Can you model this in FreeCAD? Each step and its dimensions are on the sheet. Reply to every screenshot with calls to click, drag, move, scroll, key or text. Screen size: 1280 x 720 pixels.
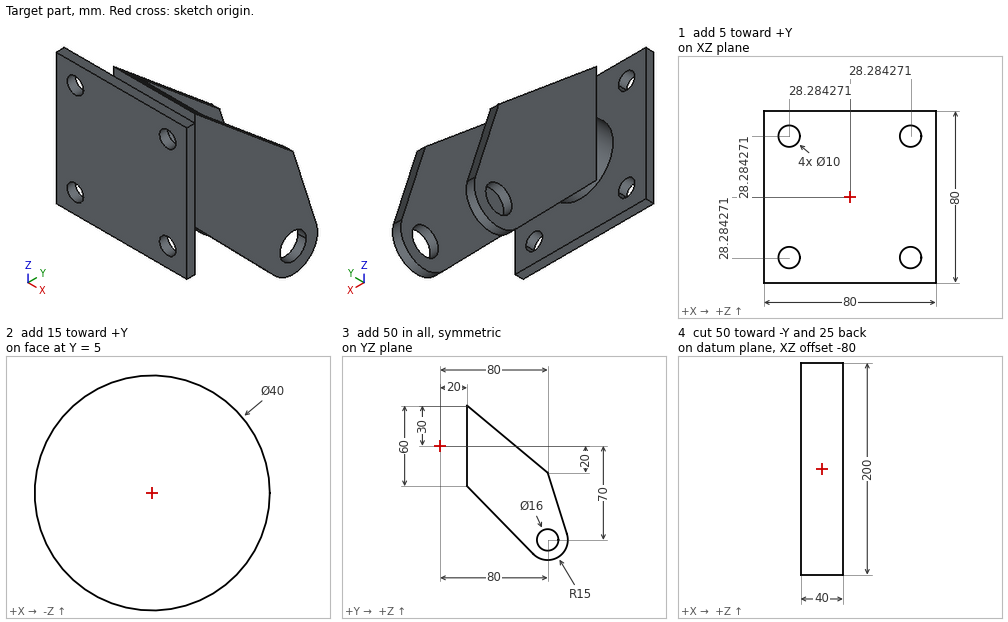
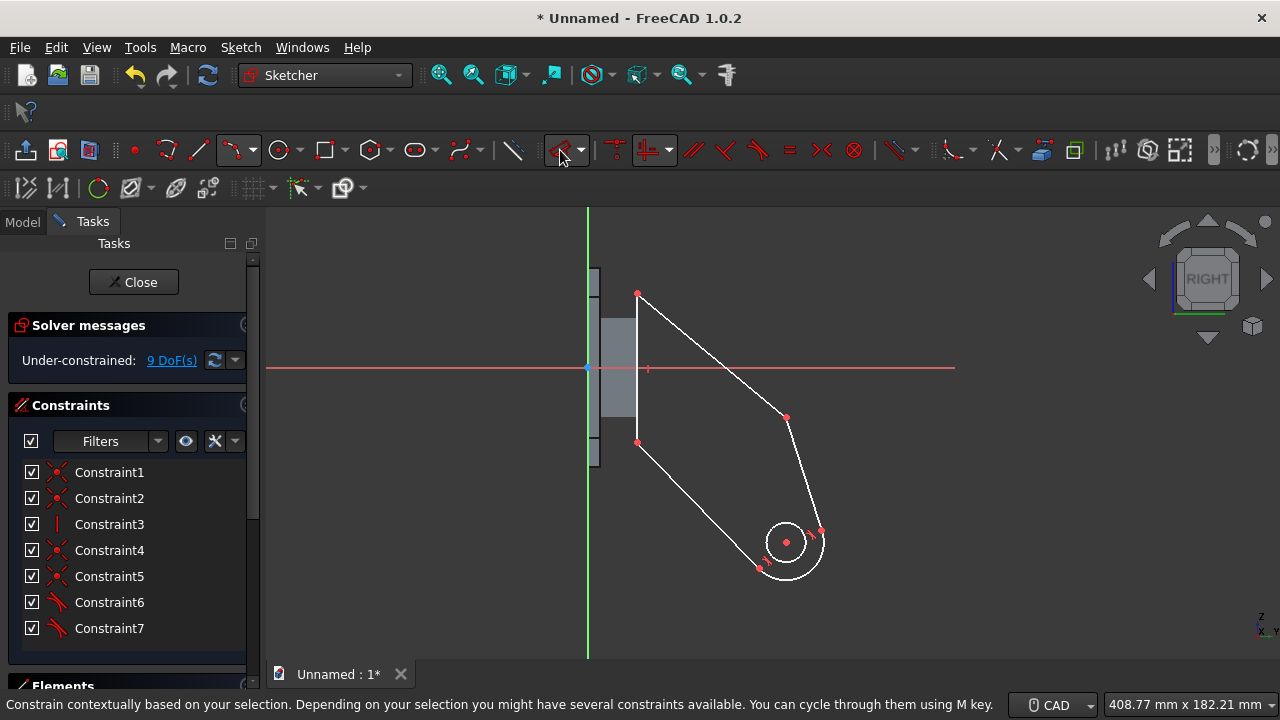
click(786, 580)
click(786, 612)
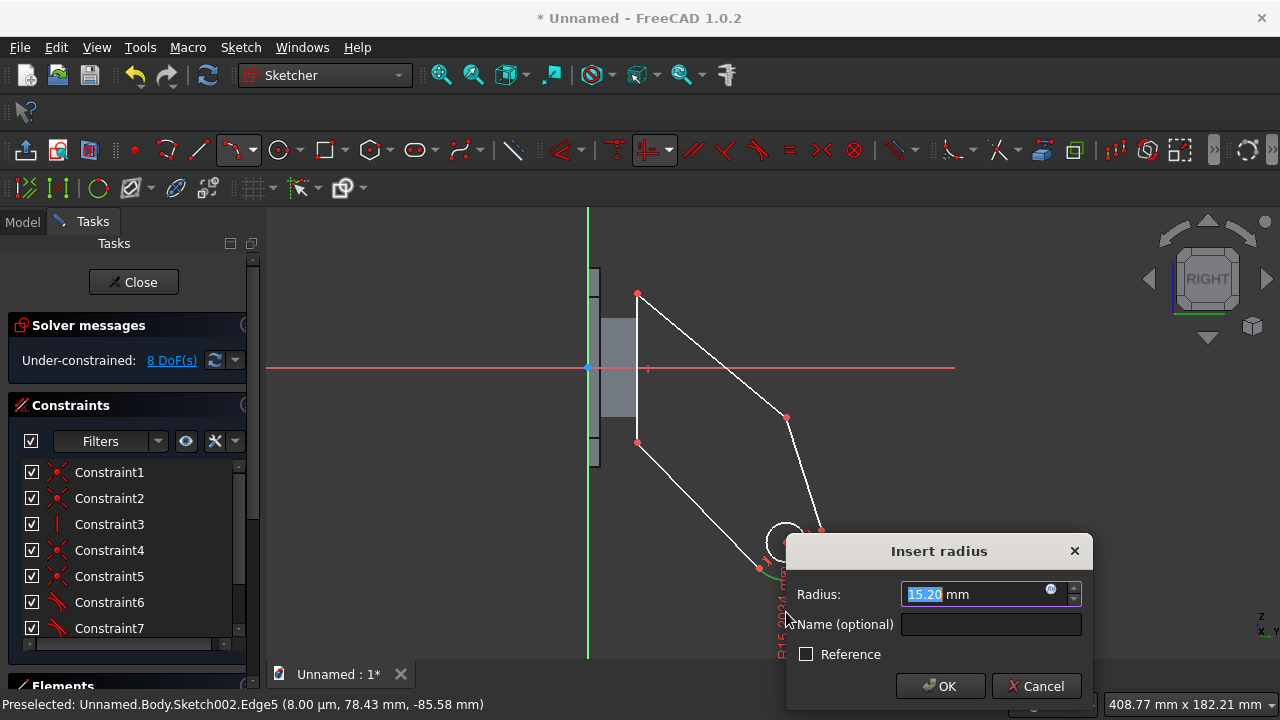
text(15)
key(Return)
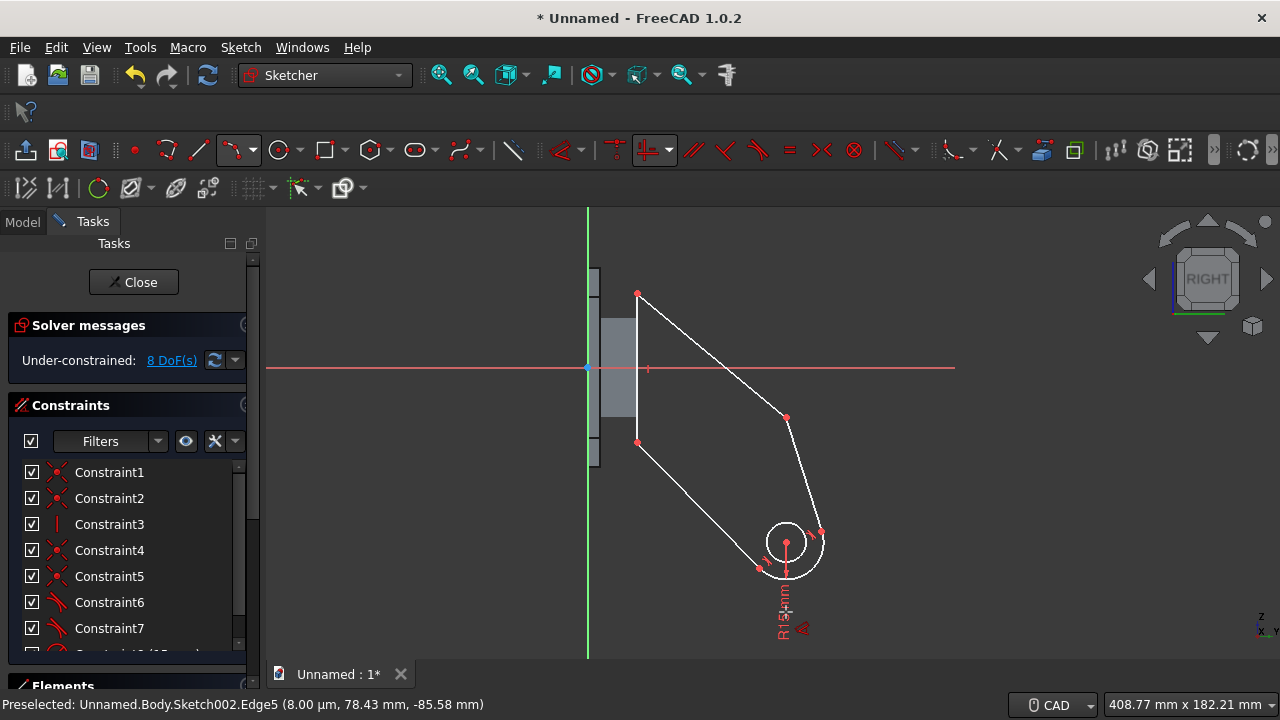
click(800, 528)
click(836, 527)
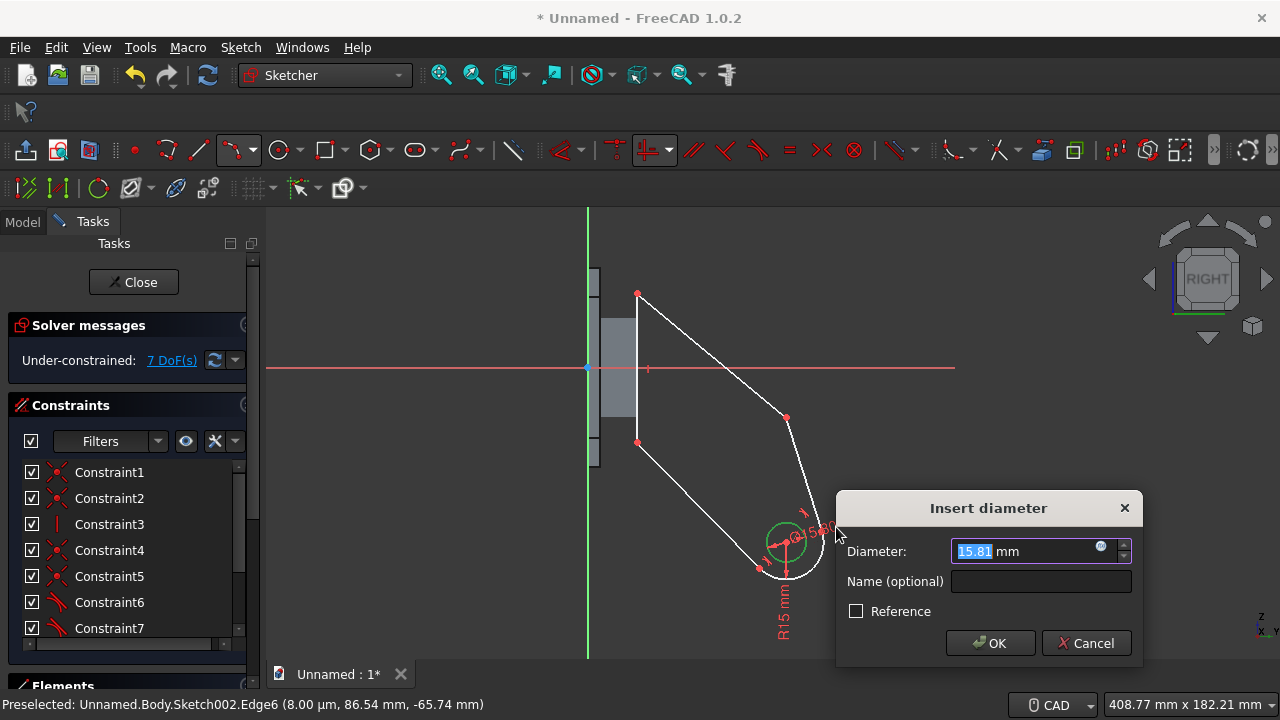
text(16)
key(Return)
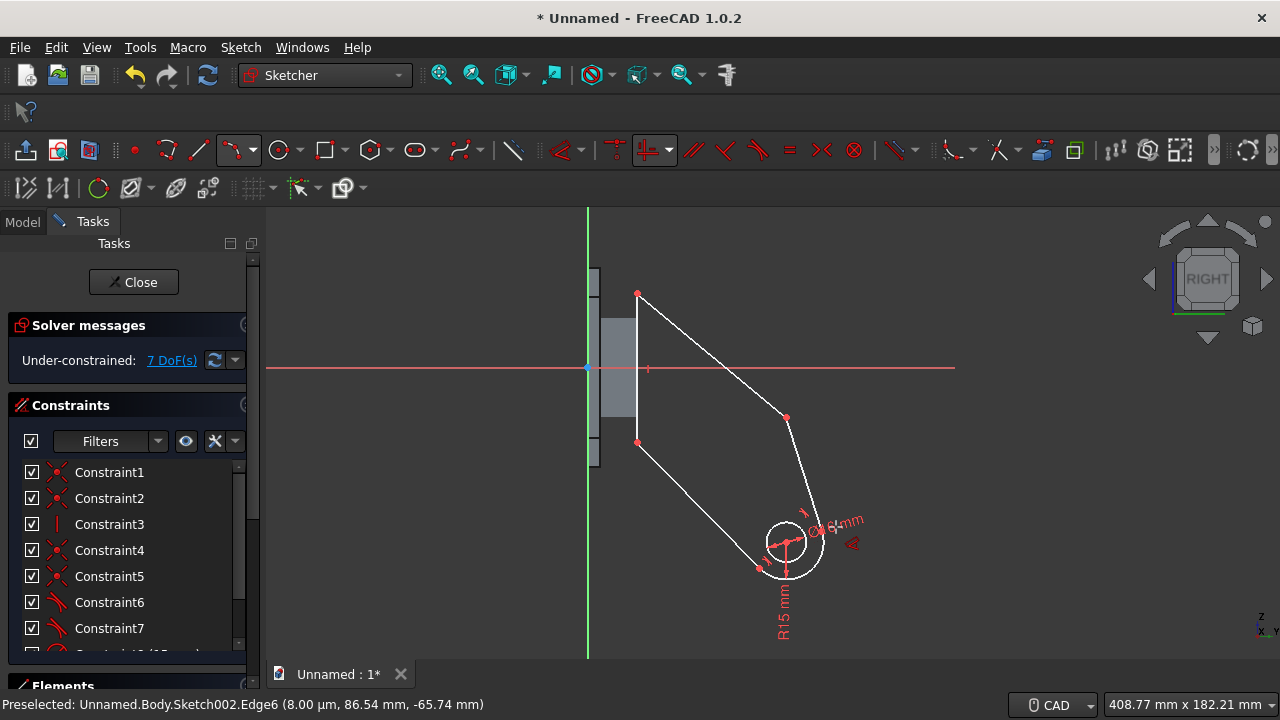
click(637, 339)
click(603, 334)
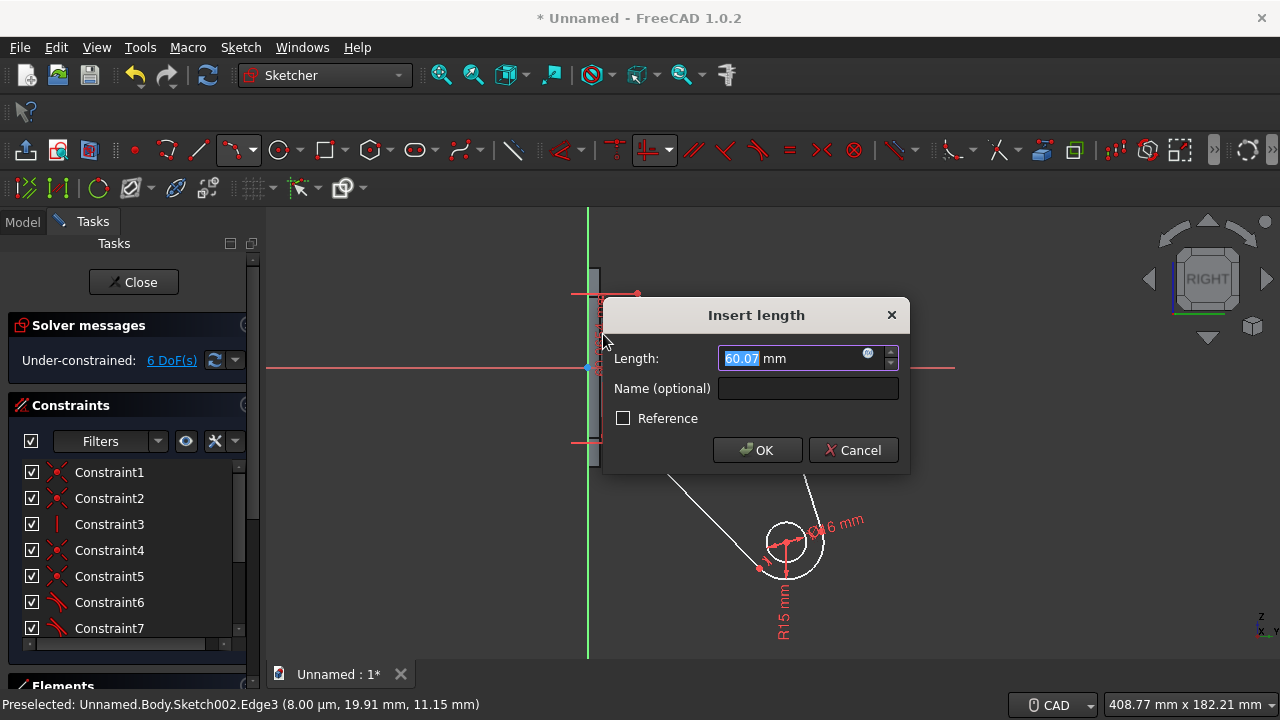
text(60)
key(Return)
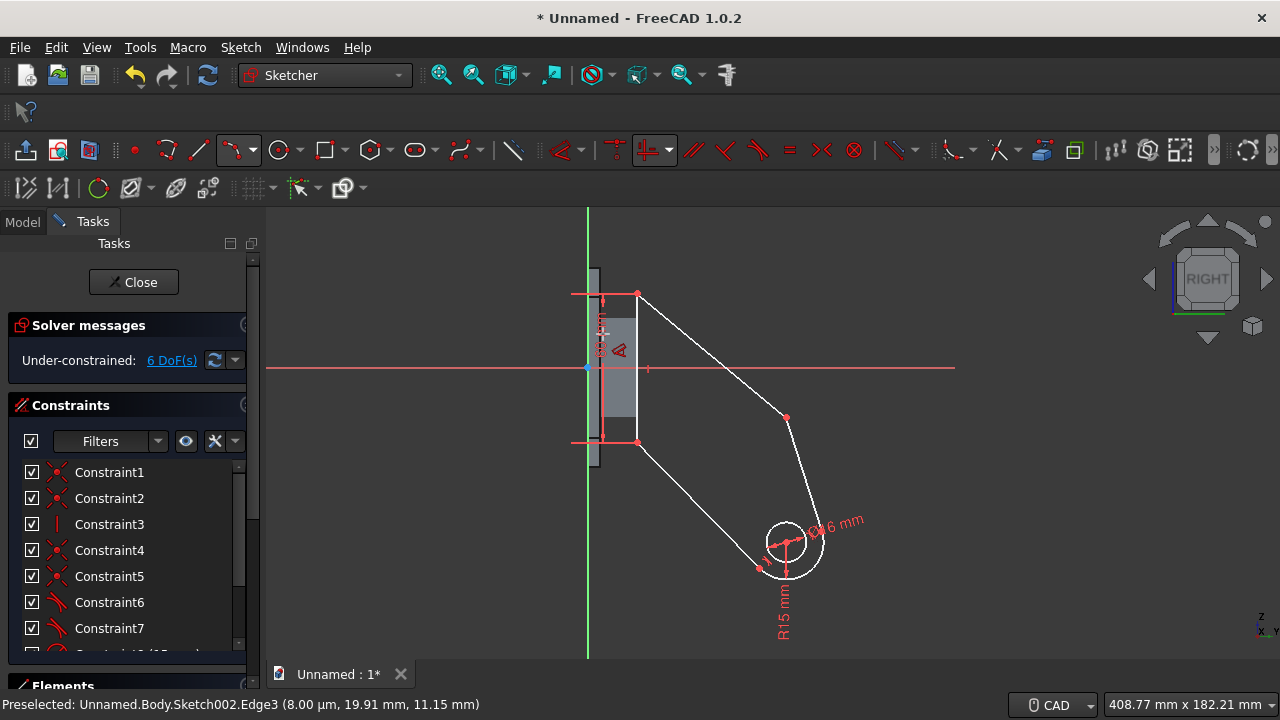
click(786, 542)
click(687, 576)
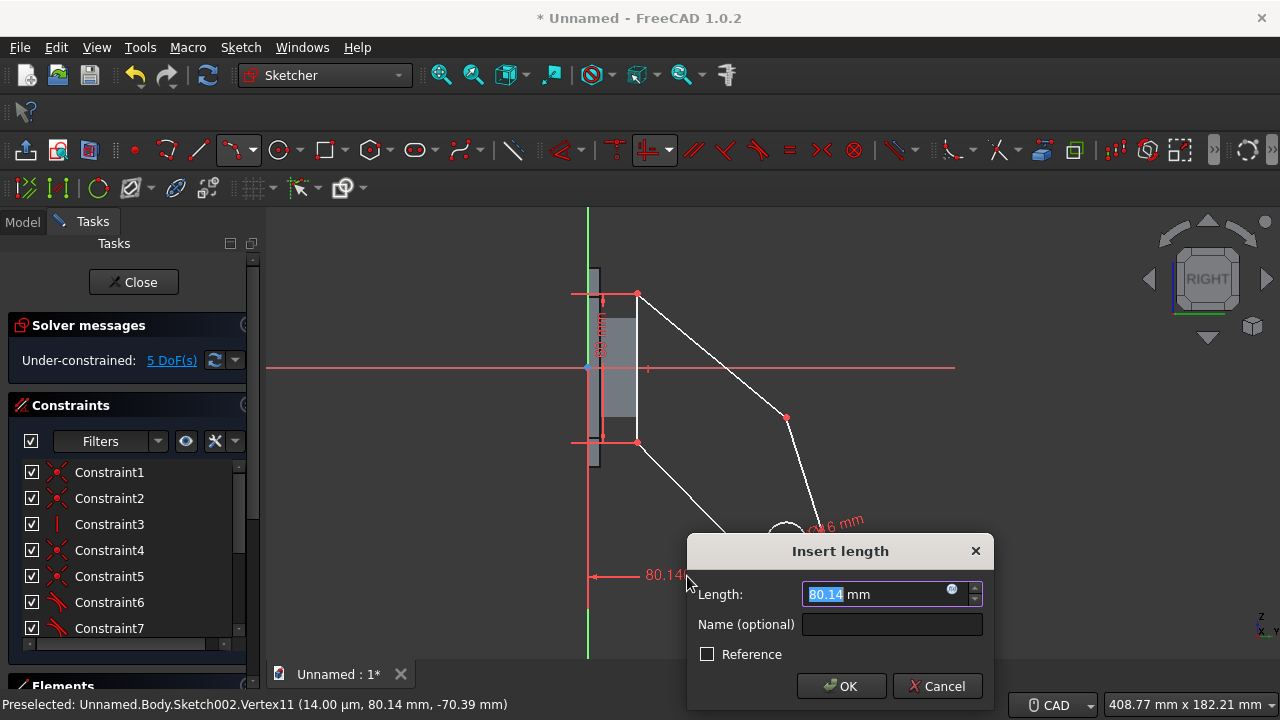
text(80)
key(Return)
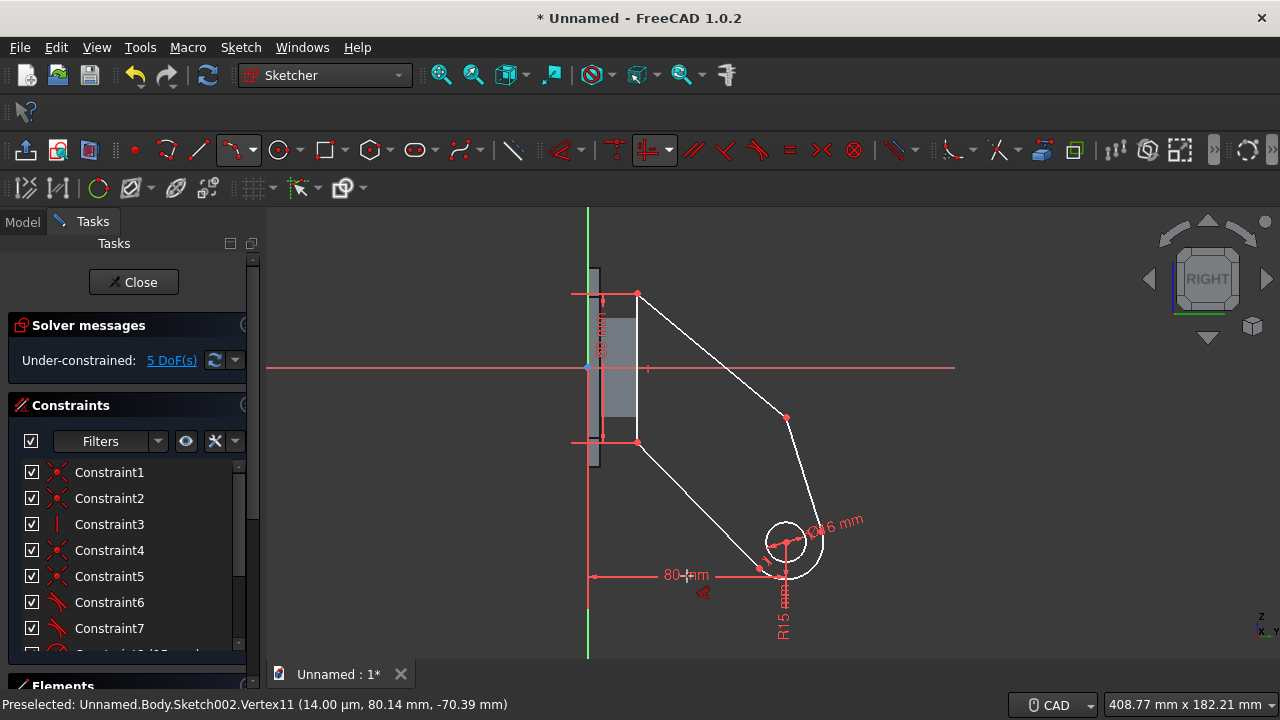
click(786, 542)
click(554, 455)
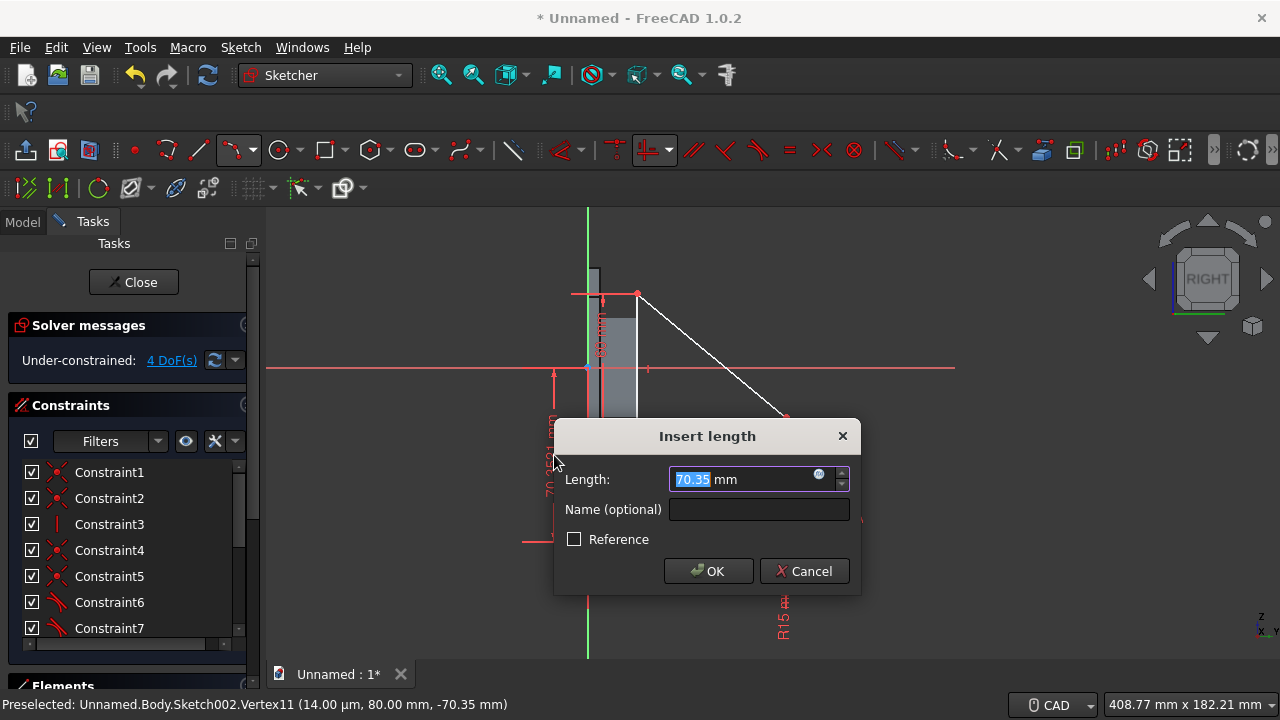
text(70)
key(Return)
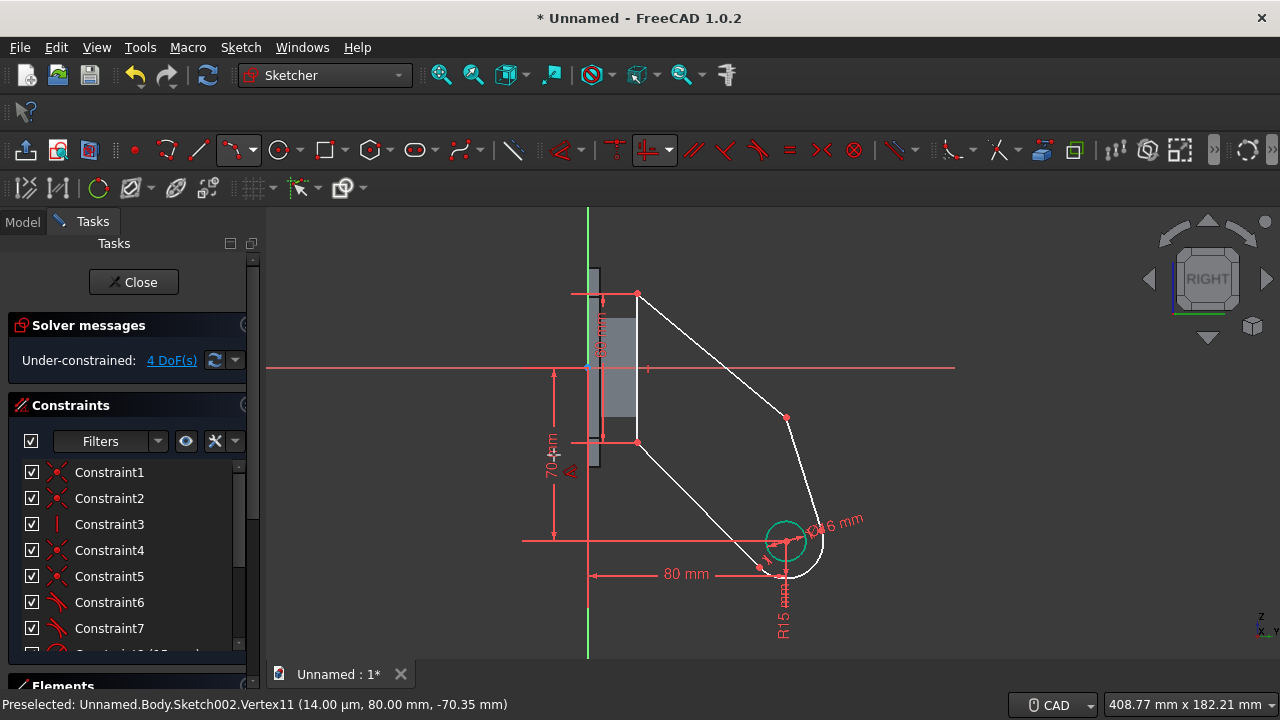
click(786, 418)
click(732, 334)